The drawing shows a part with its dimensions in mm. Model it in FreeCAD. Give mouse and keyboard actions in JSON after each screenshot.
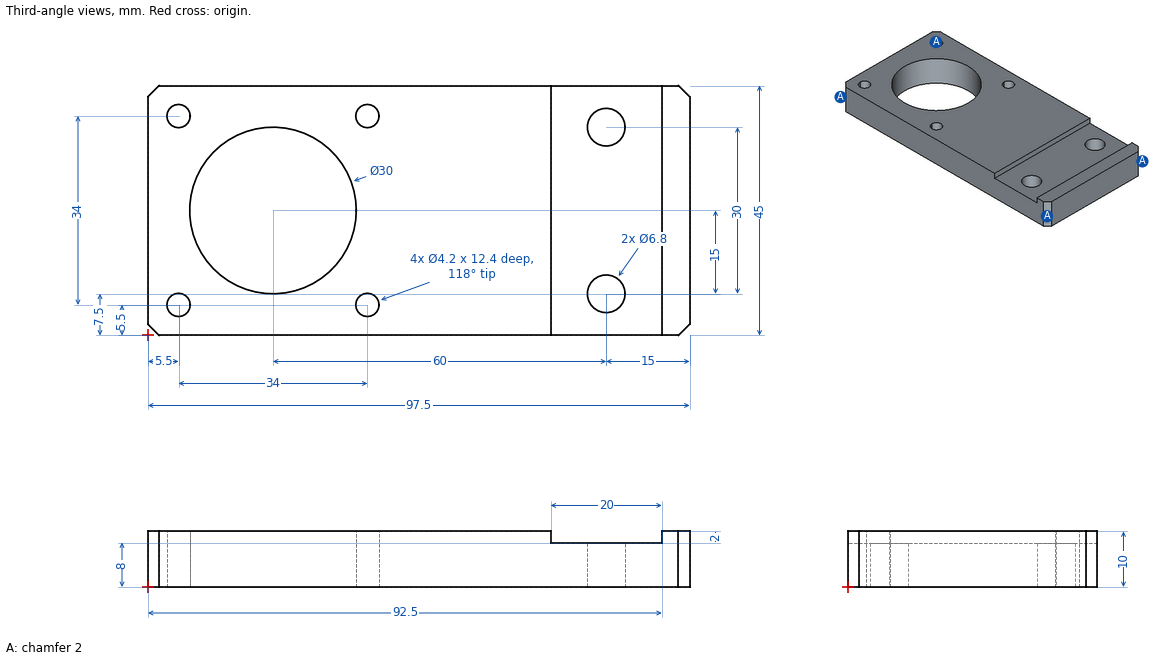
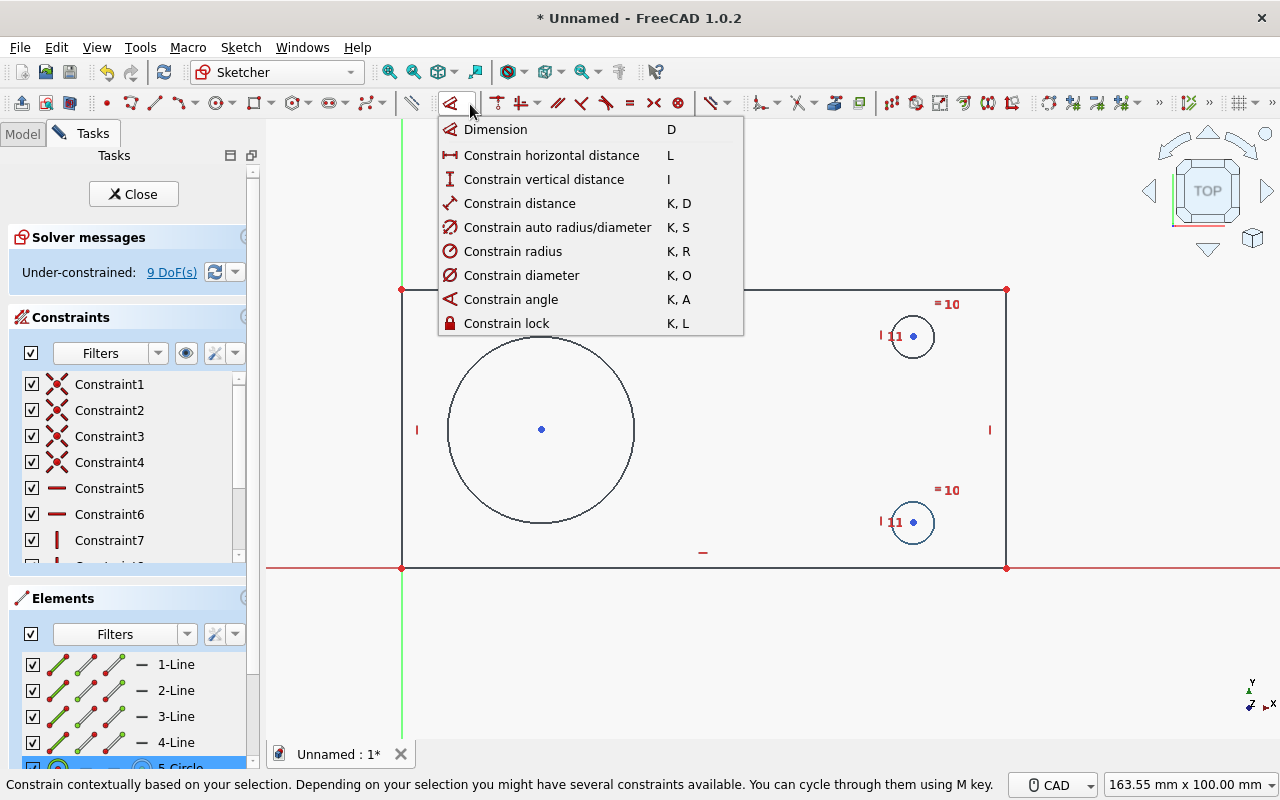
{"action": "left_click", "coordinate": [591, 275]}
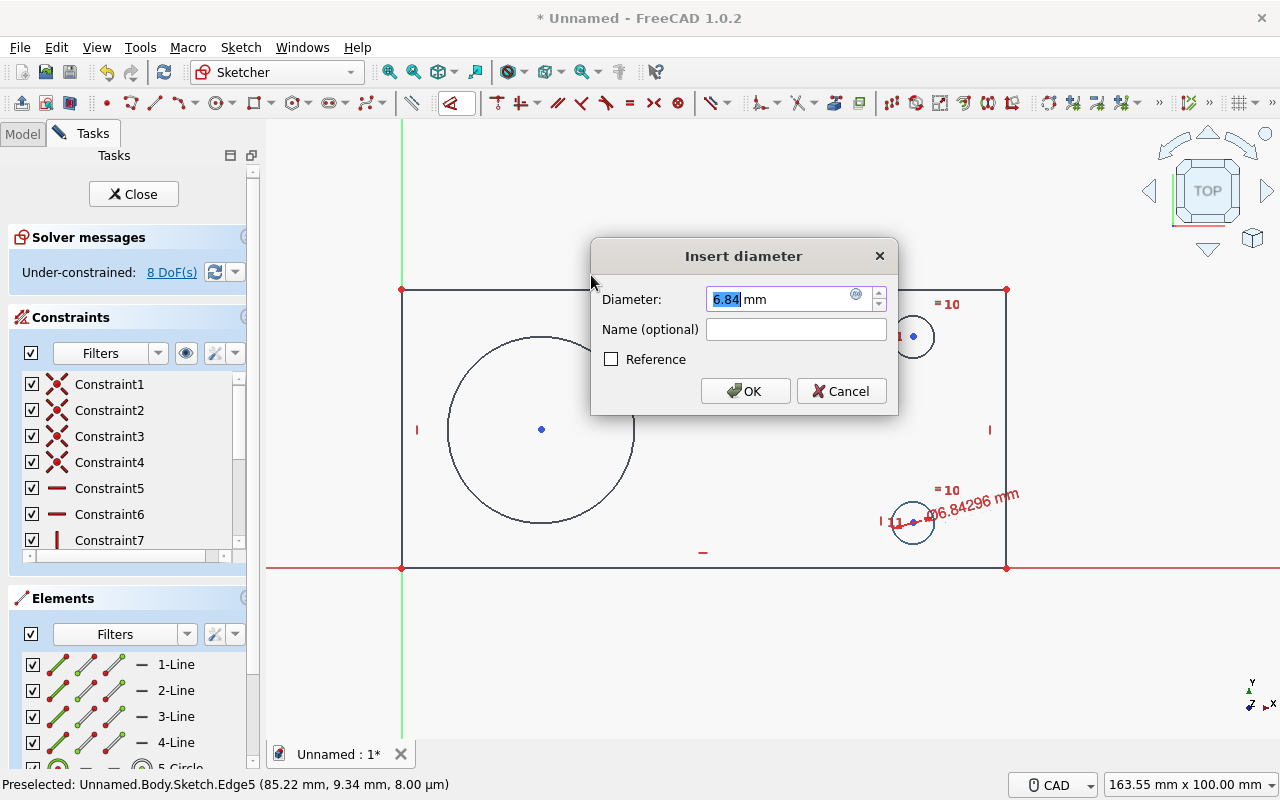
{"action": "type", "text": "6.8"}
{"action": "key", "text": "Return"}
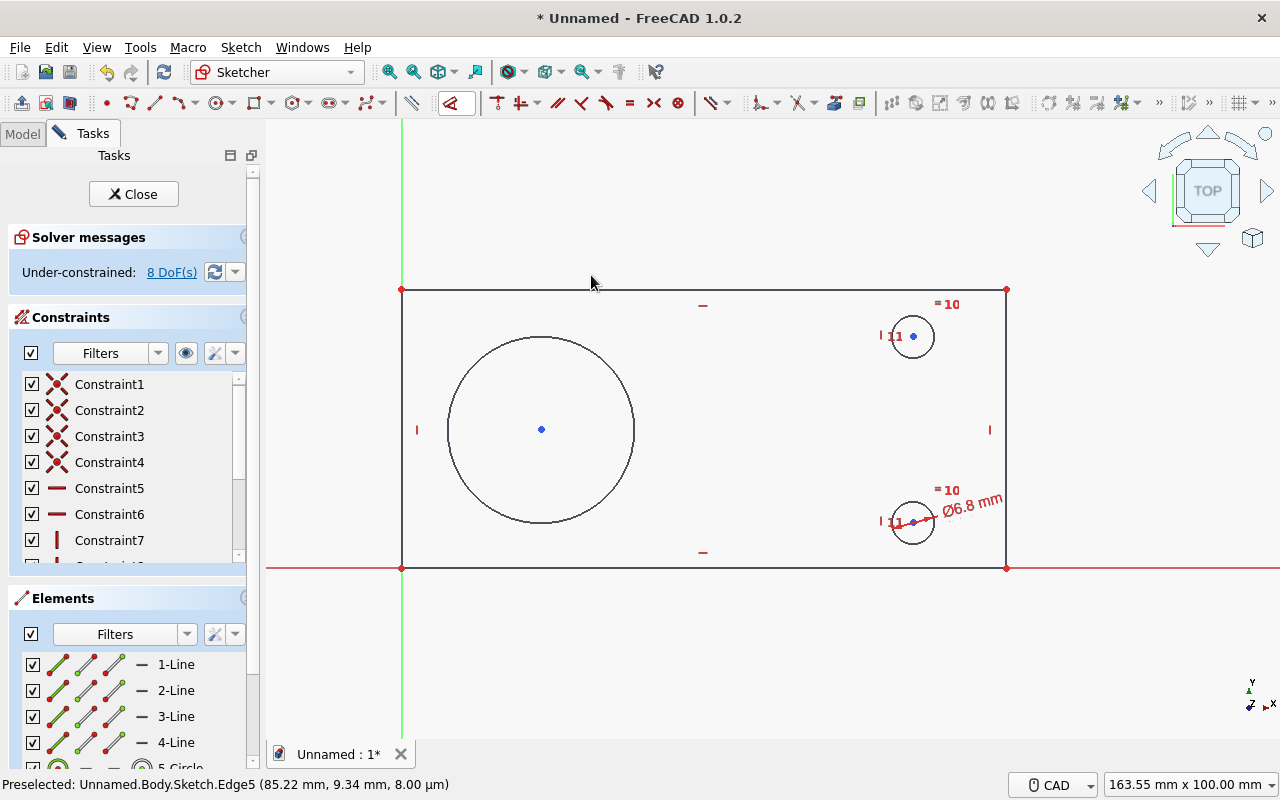
{"action": "left_click", "coordinate": [607, 364]}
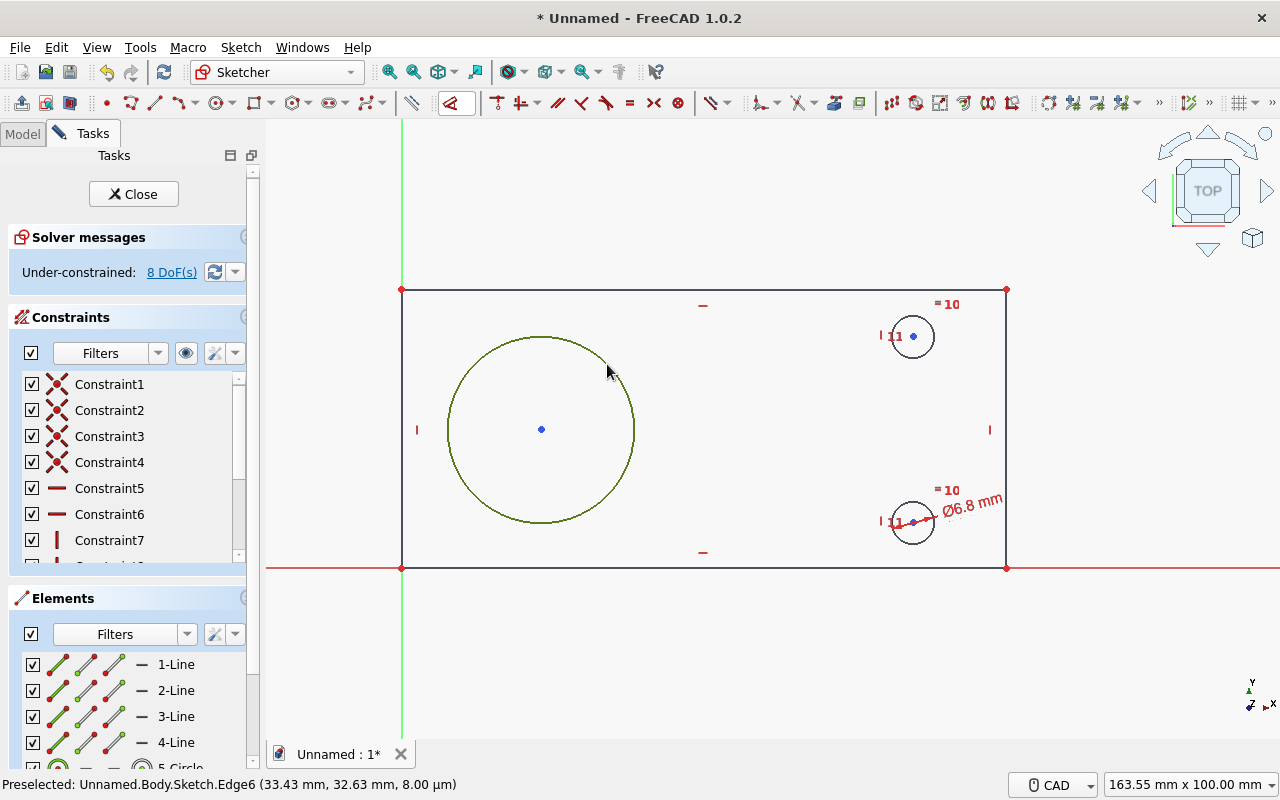
{"action": "key", "text": "k o"}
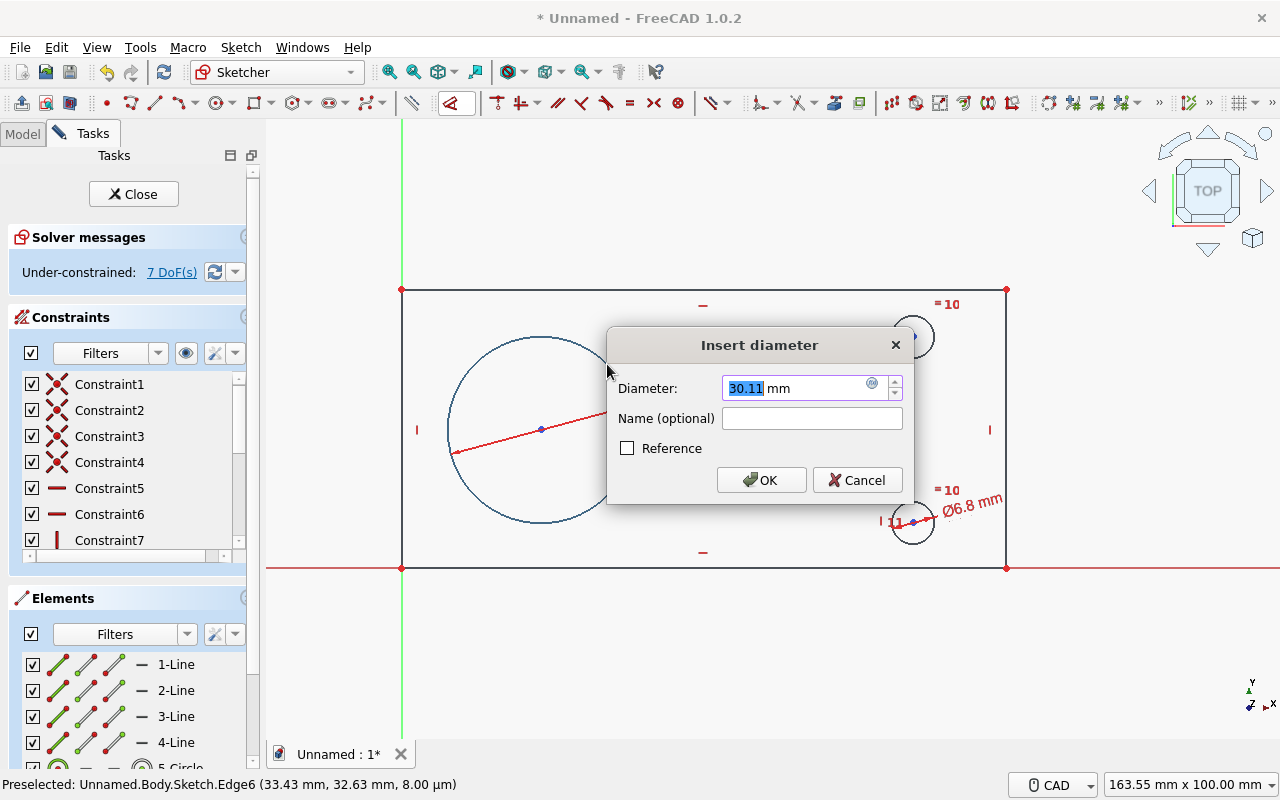
{"action": "type", "text": "30"}
{"action": "key", "text": "Return"}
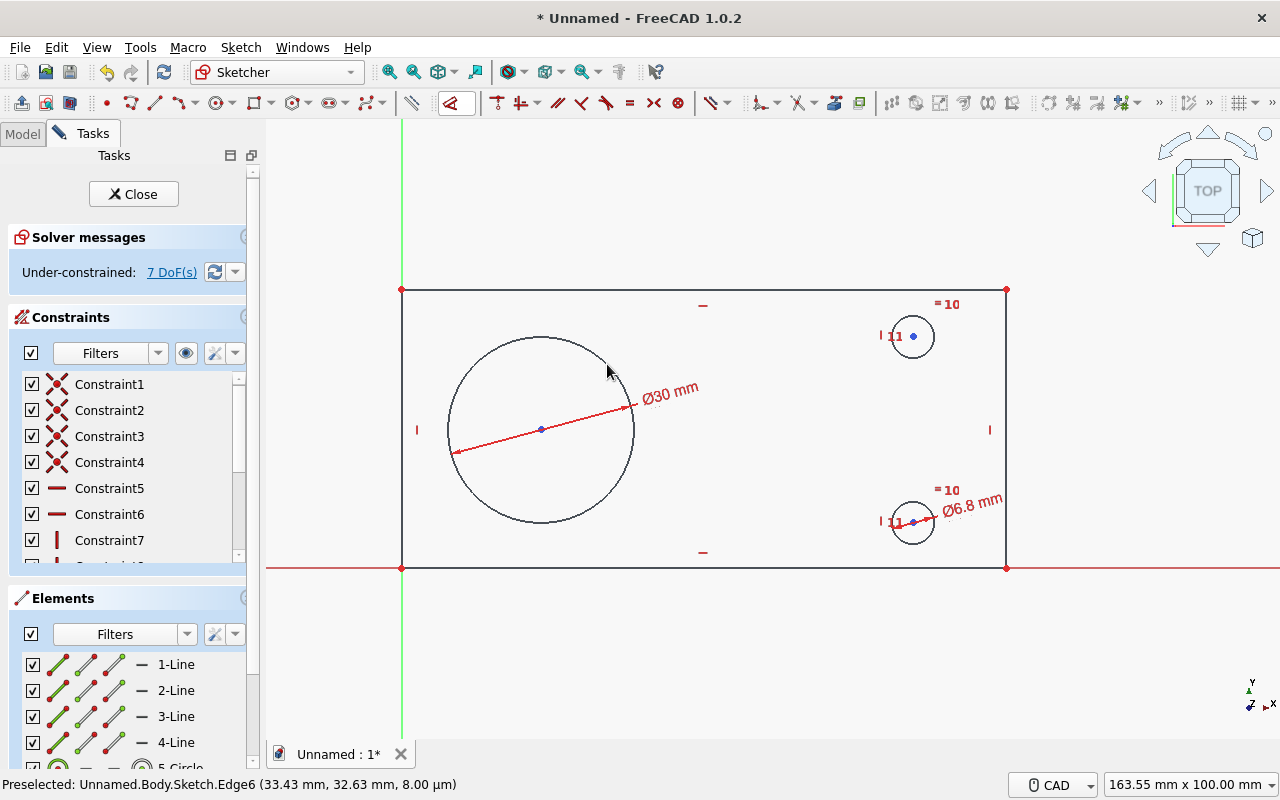
{"action": "left_click", "coordinate": [1006, 485]}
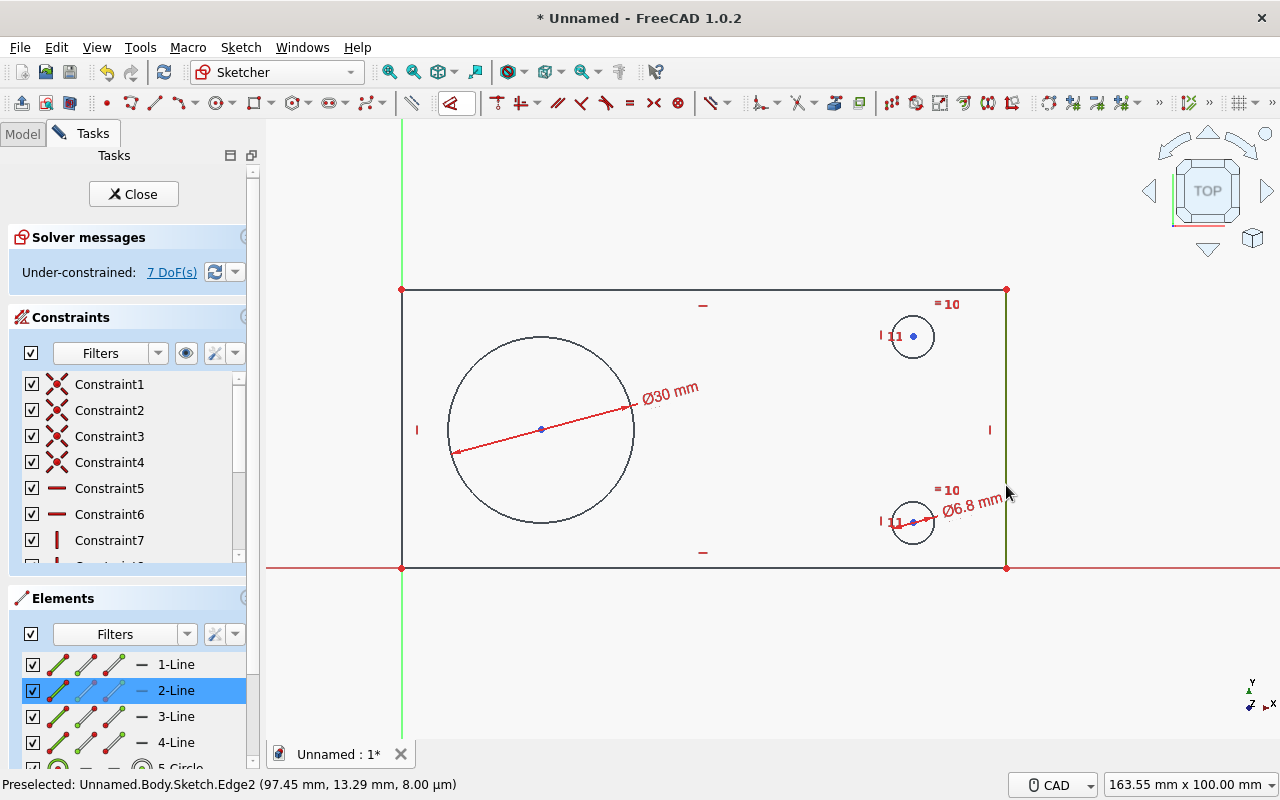
{"action": "key", "text": "i"}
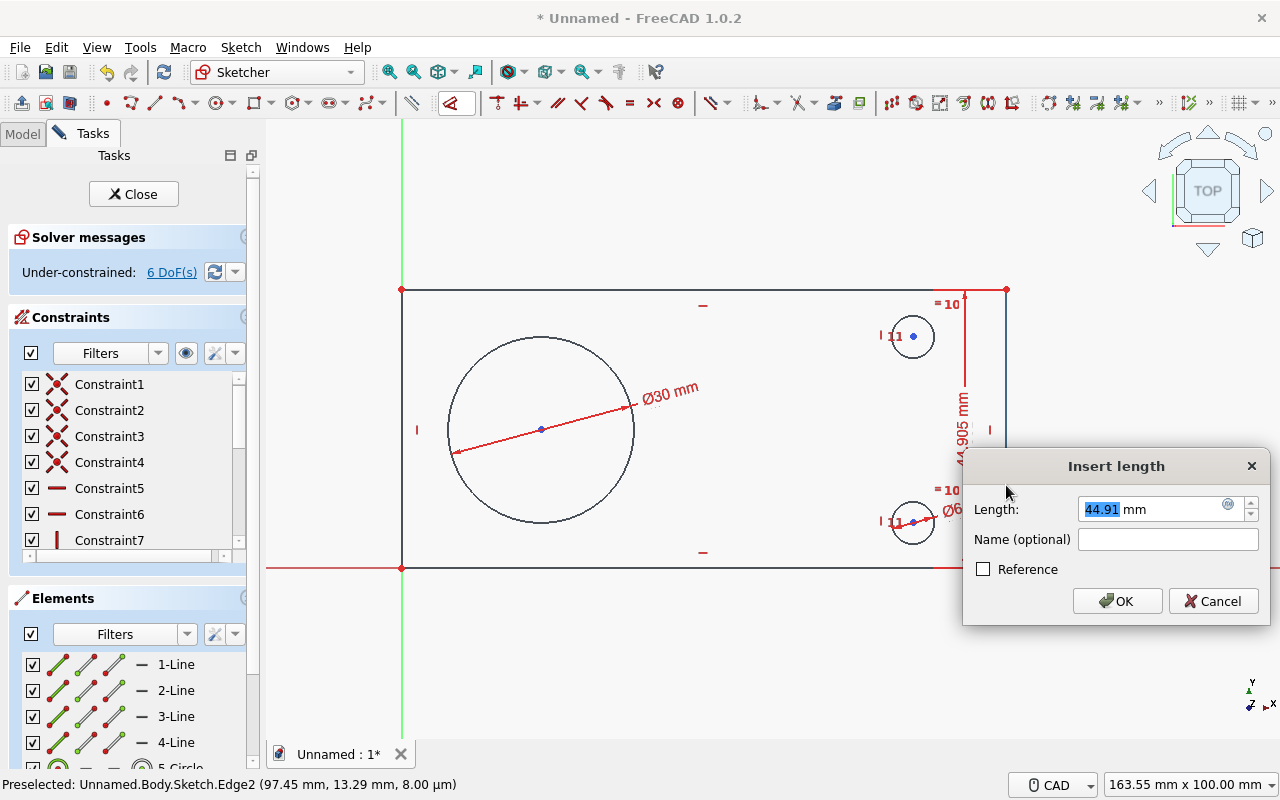
{"action": "type", "text": "45"}
{"action": "key", "text": "Return"}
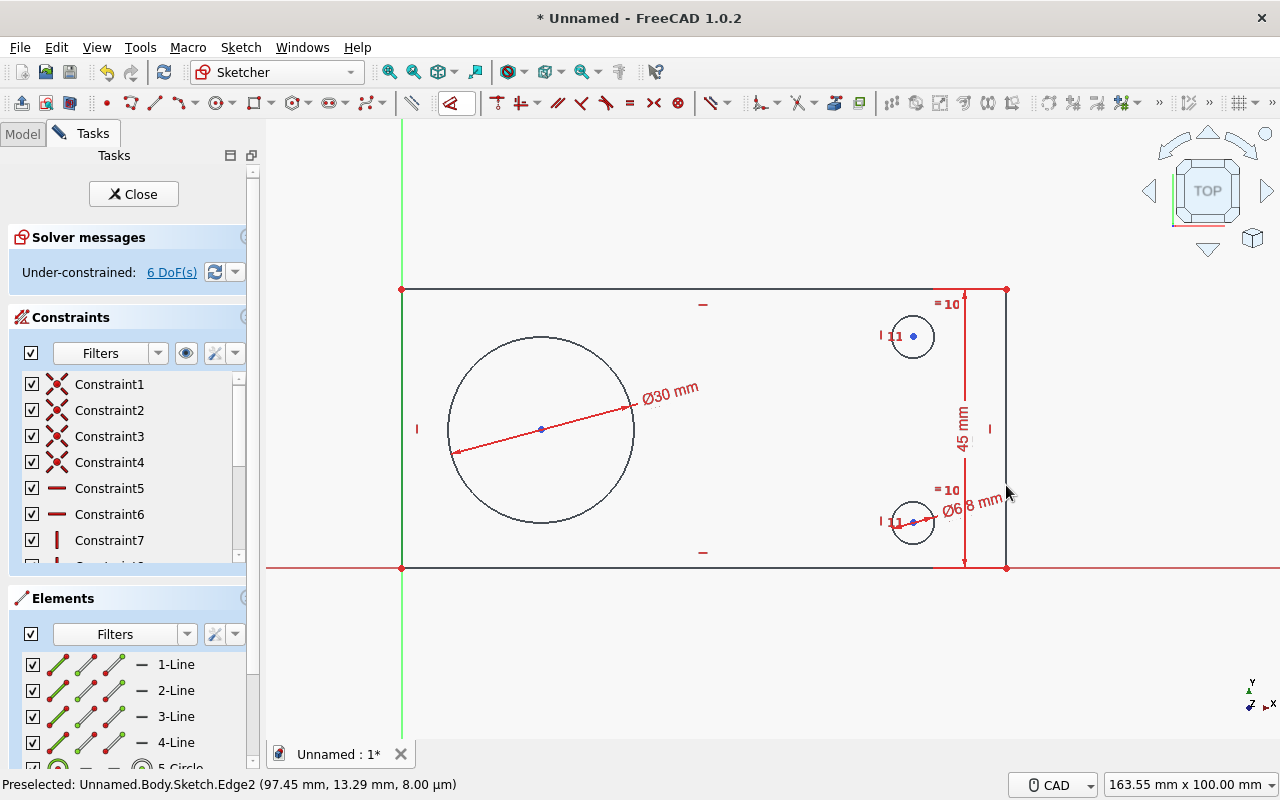
{"action": "left_click", "coordinate": [913, 523]}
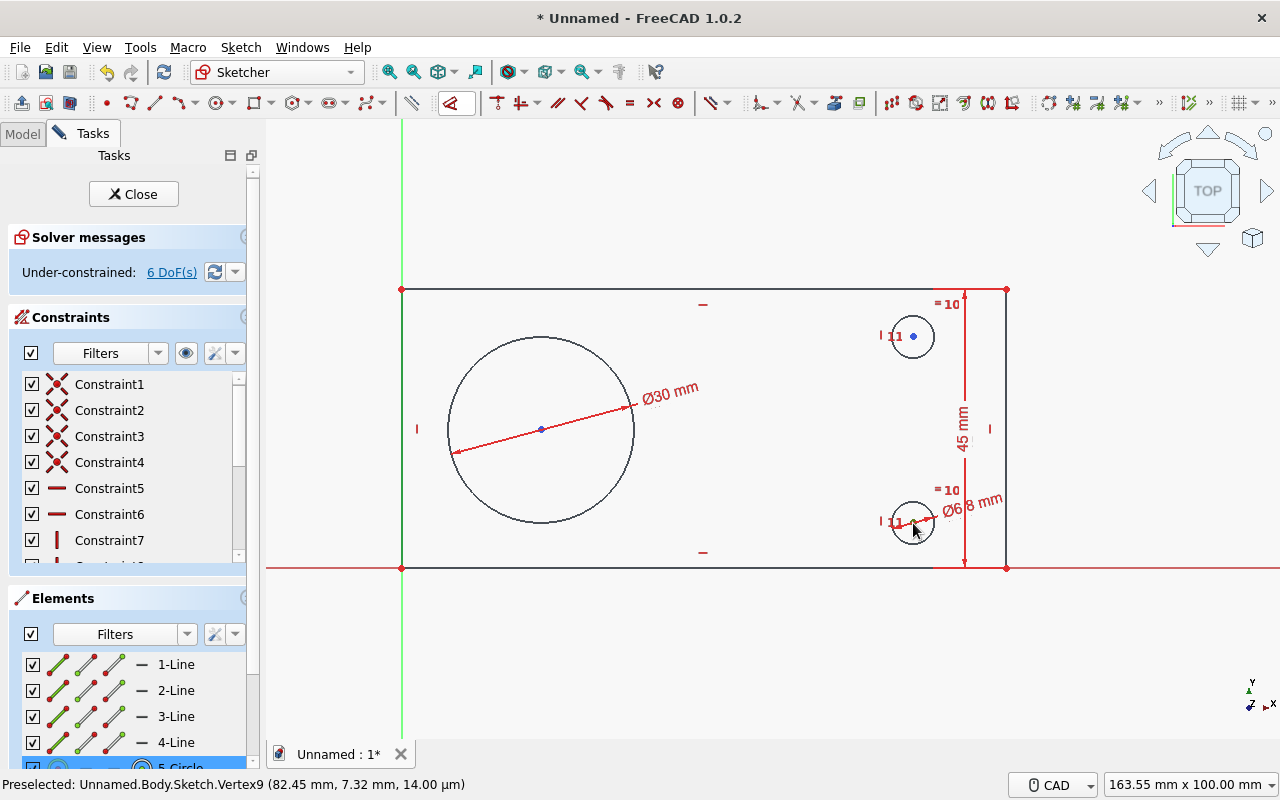
{"action": "key", "text": "i"}